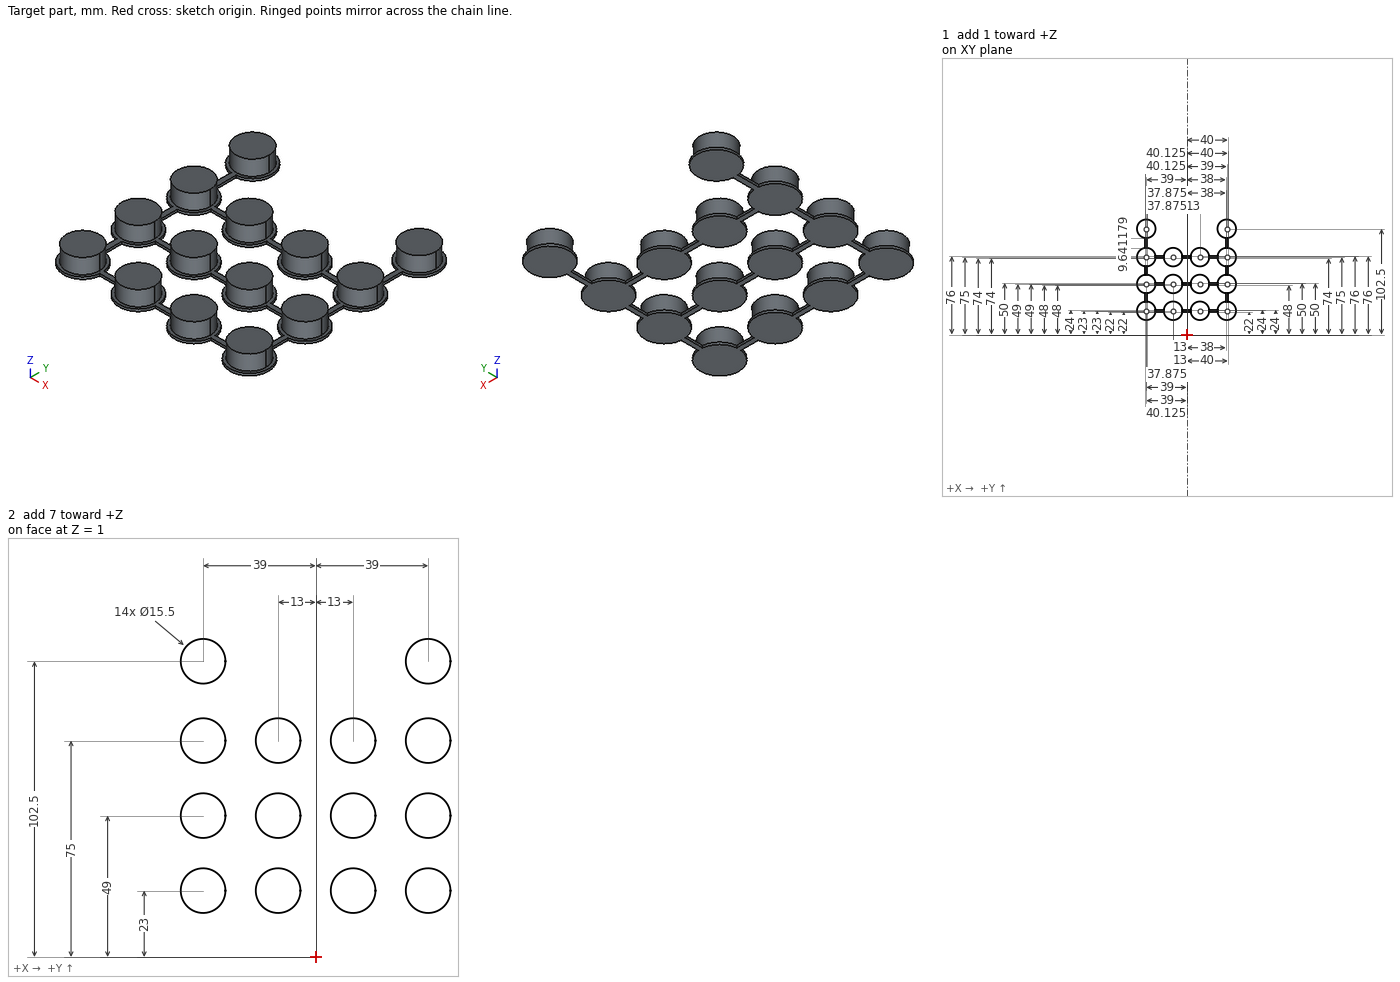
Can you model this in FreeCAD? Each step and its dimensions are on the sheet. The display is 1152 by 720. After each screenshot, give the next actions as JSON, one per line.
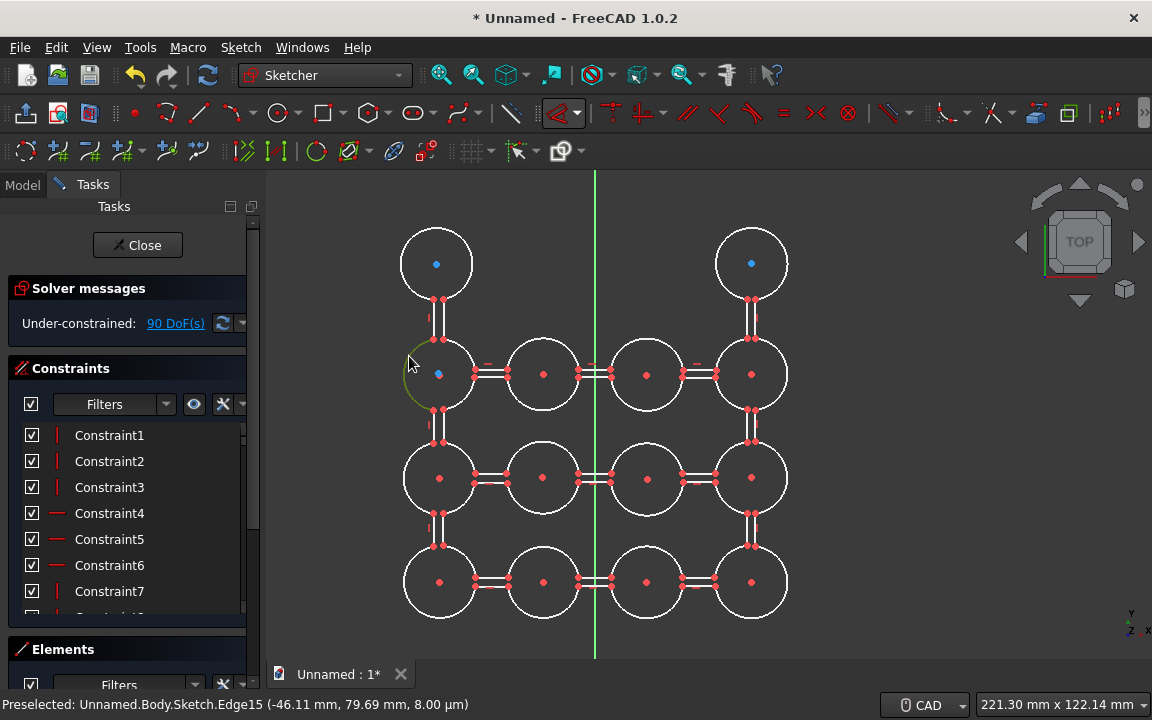
{"action": "left_click", "coordinate": [457, 405]}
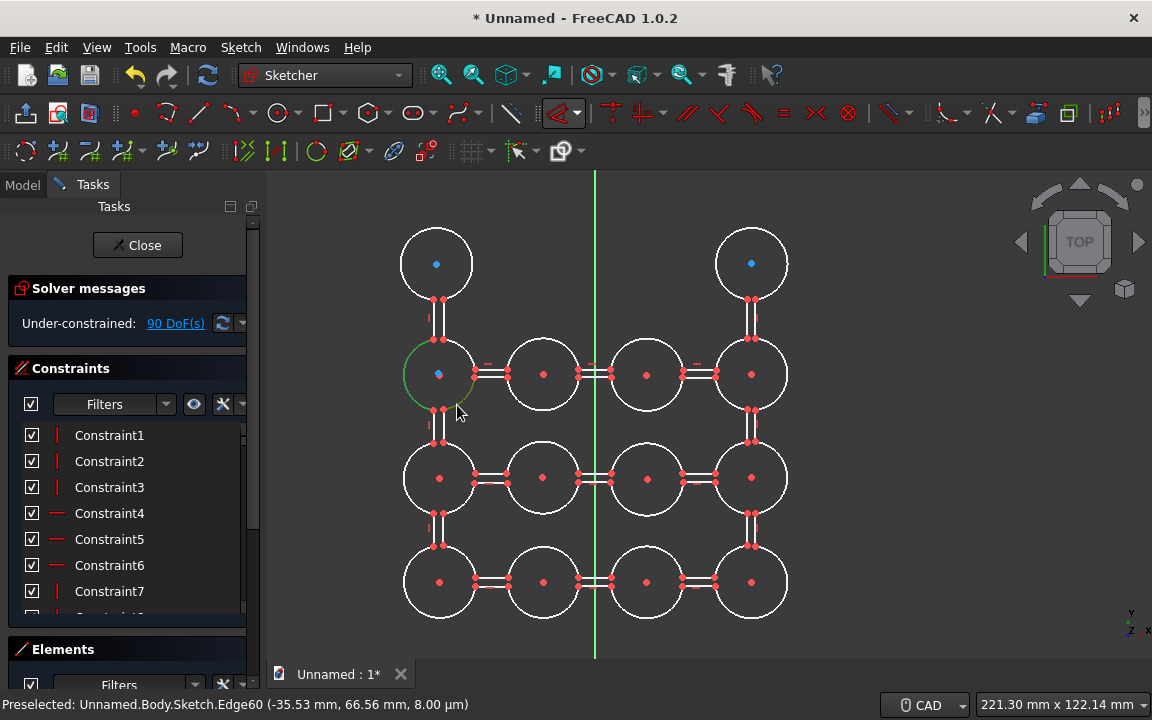
{"action": "left_click", "coordinate": [612, 114]}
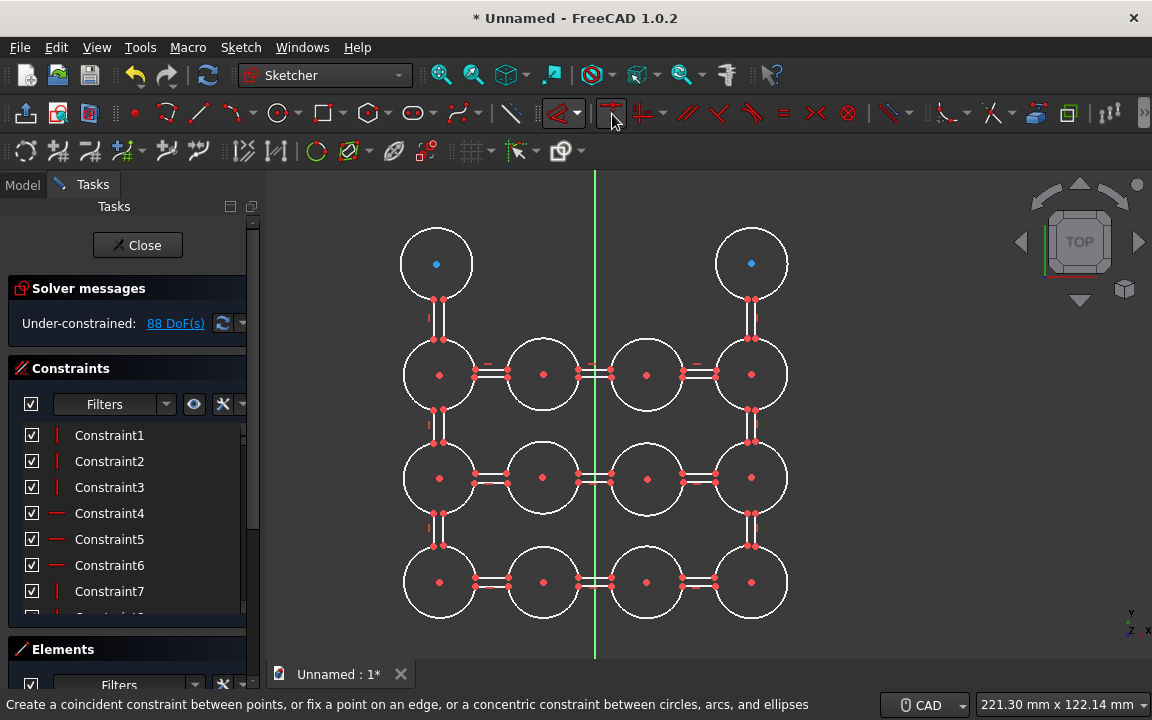
{"action": "left_click", "coordinate": [409, 356]}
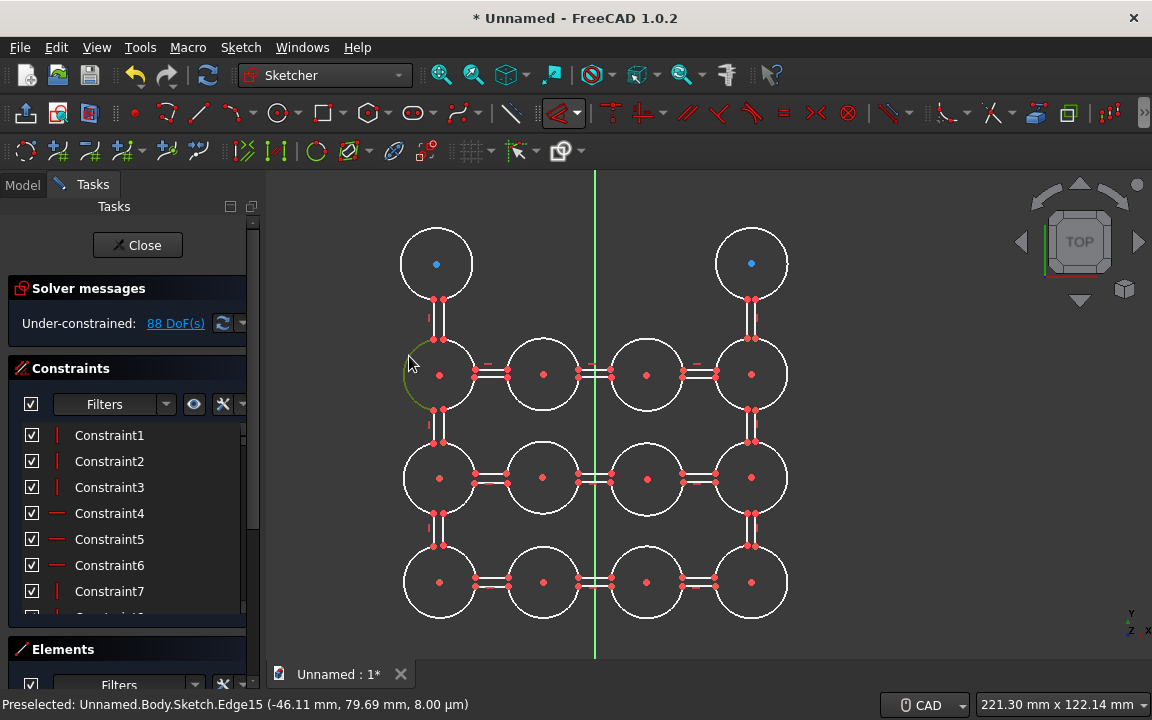
{"action": "left_click", "coordinate": [409, 459]}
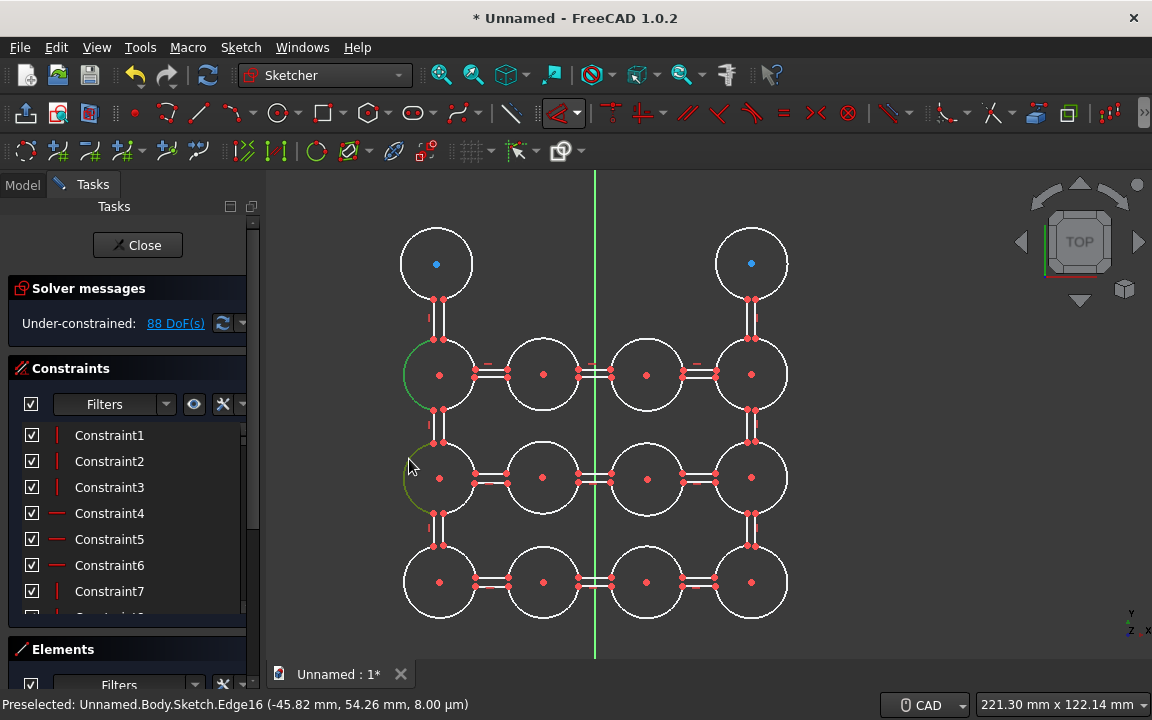
{"action": "left_click", "coordinate": [404, 579]}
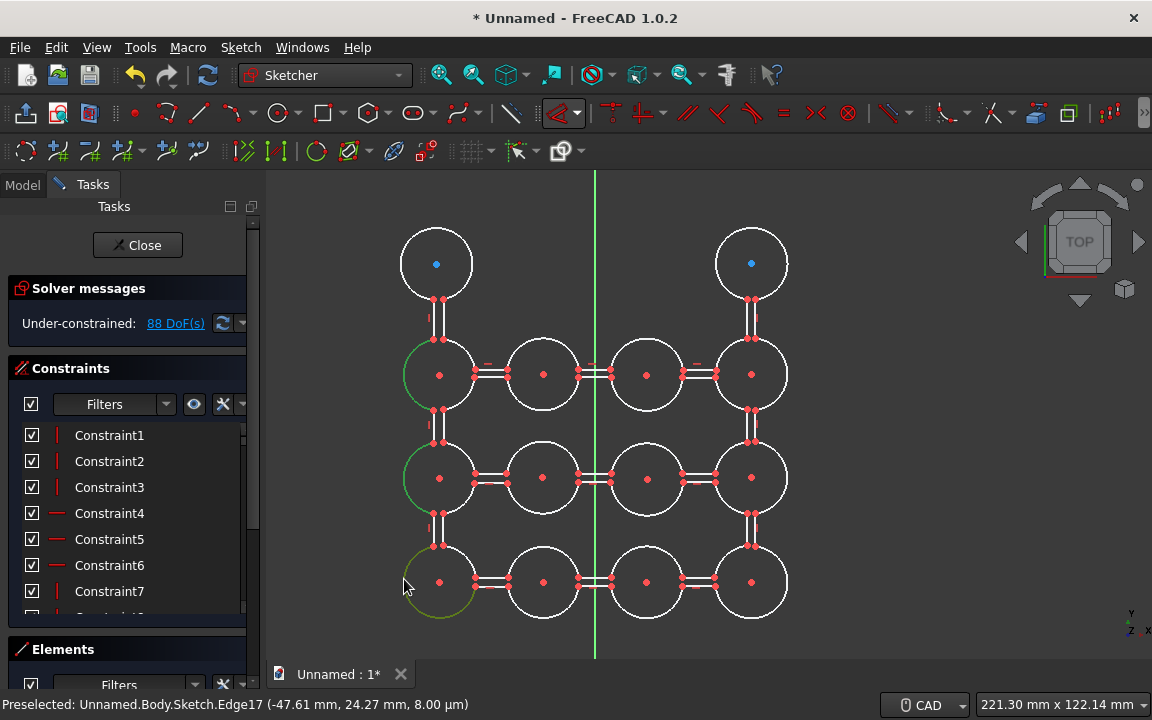
{"action": "left_click", "coordinate": [524, 612]}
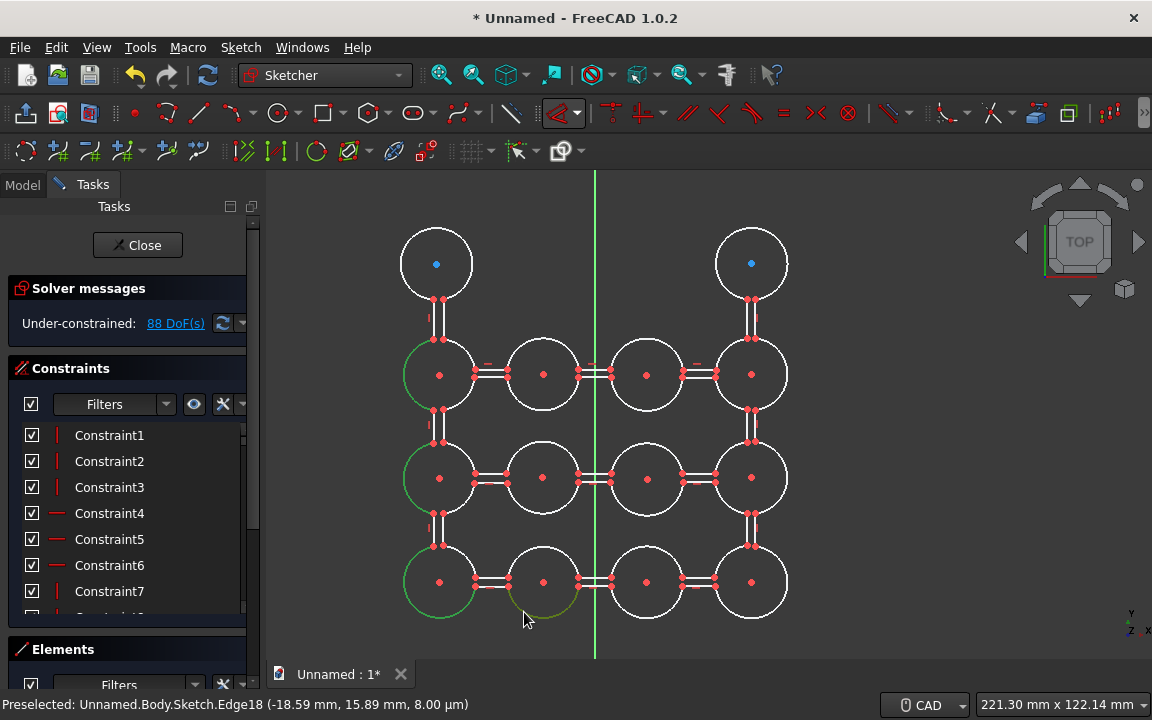
{"action": "left_click", "coordinate": [627, 612]}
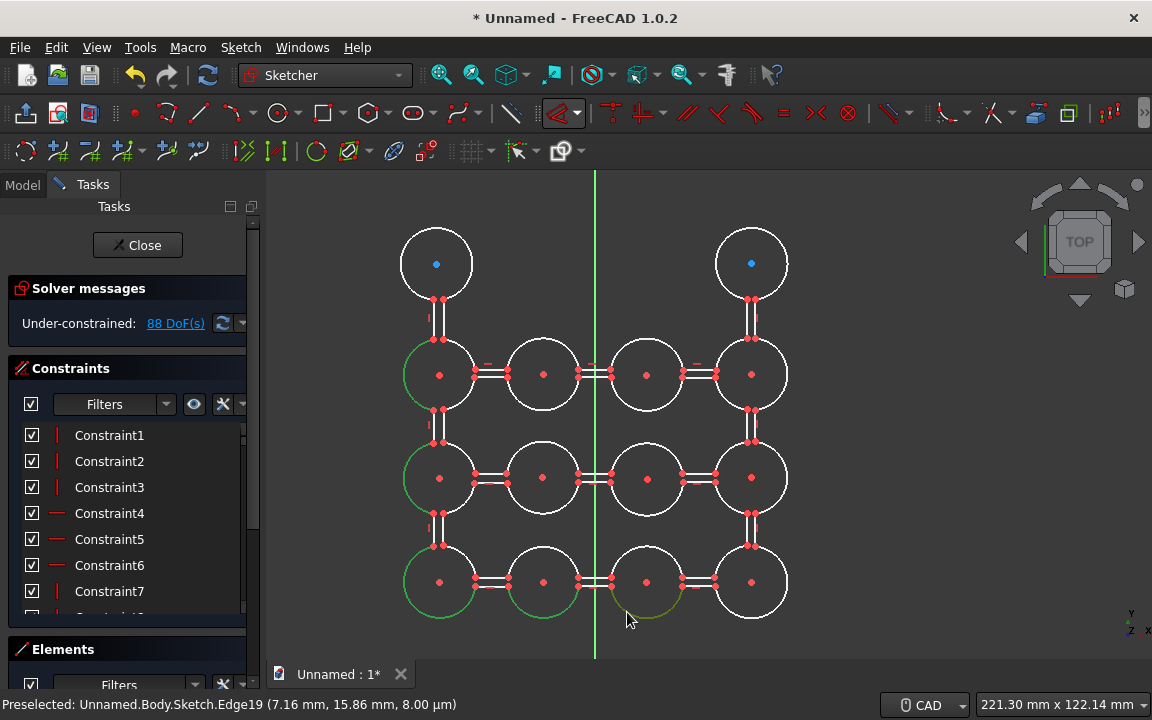
{"action": "left_click", "coordinate": [747, 618]}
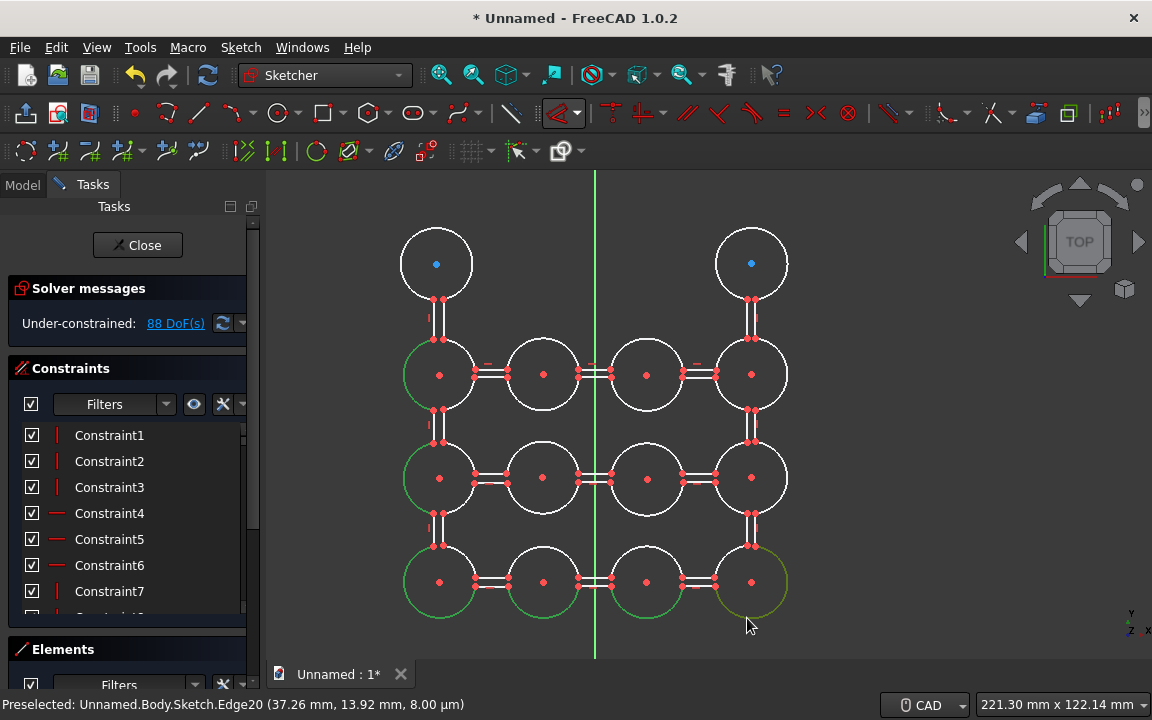
{"action": "left_click", "coordinate": [781, 498]}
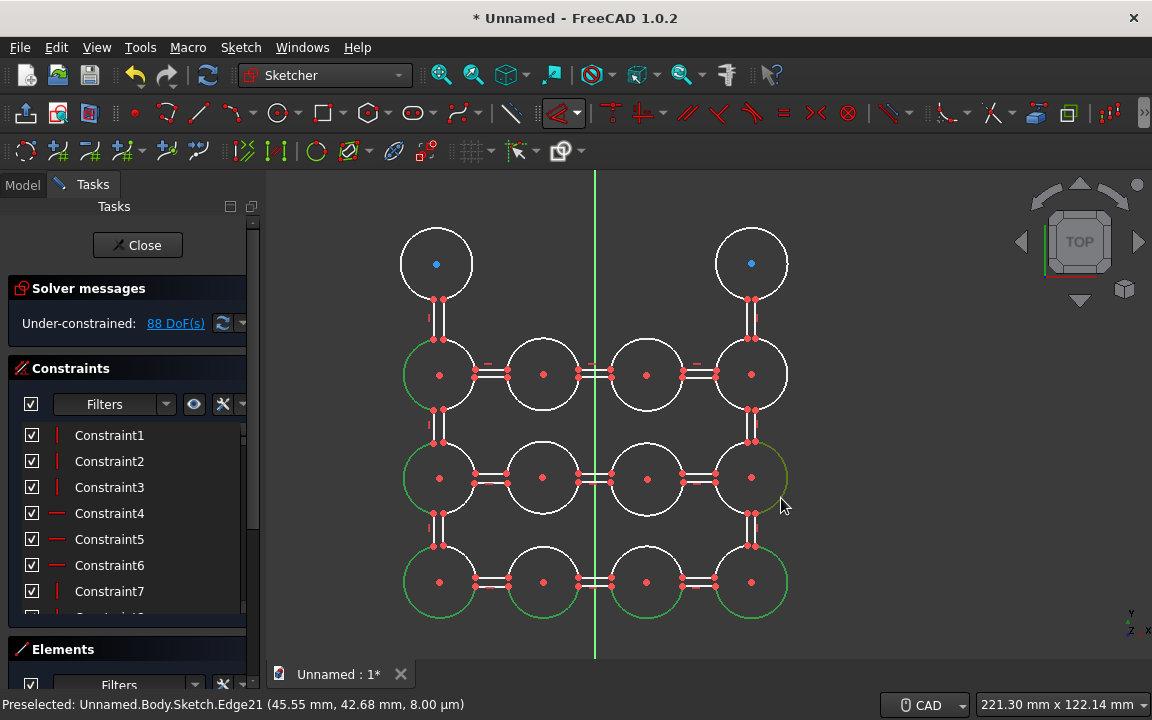
{"action": "left_click", "coordinate": [781, 394]}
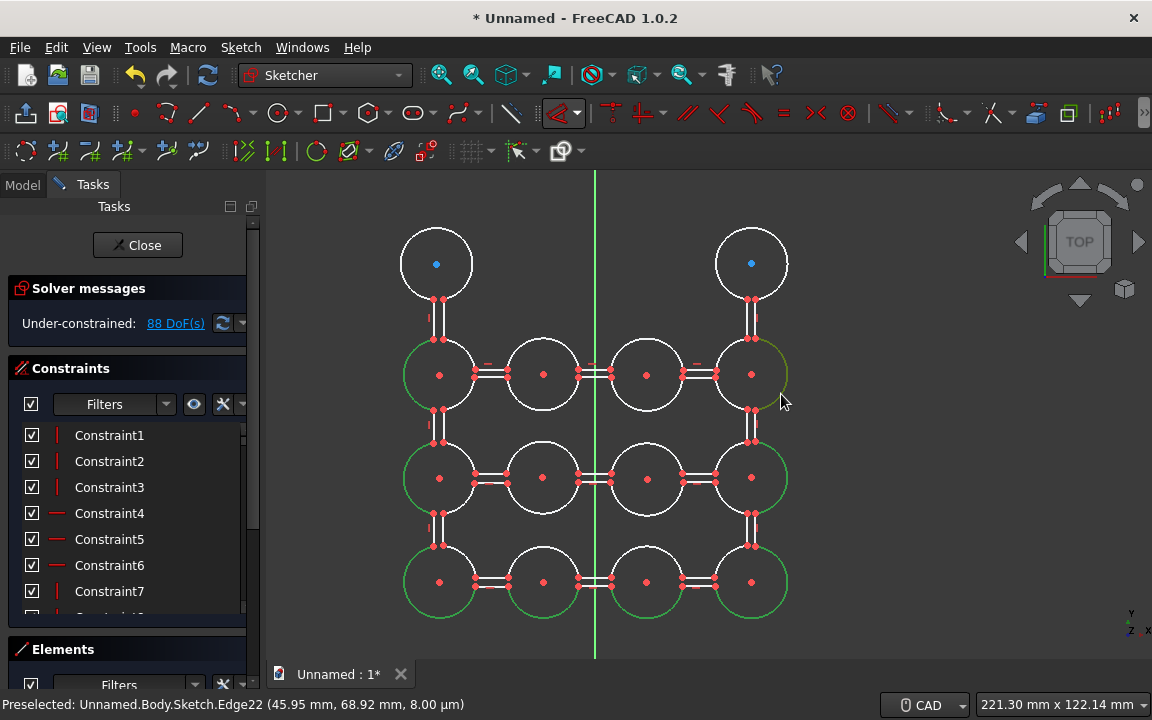
{"action": "left_click", "coordinate": [785, 251]}